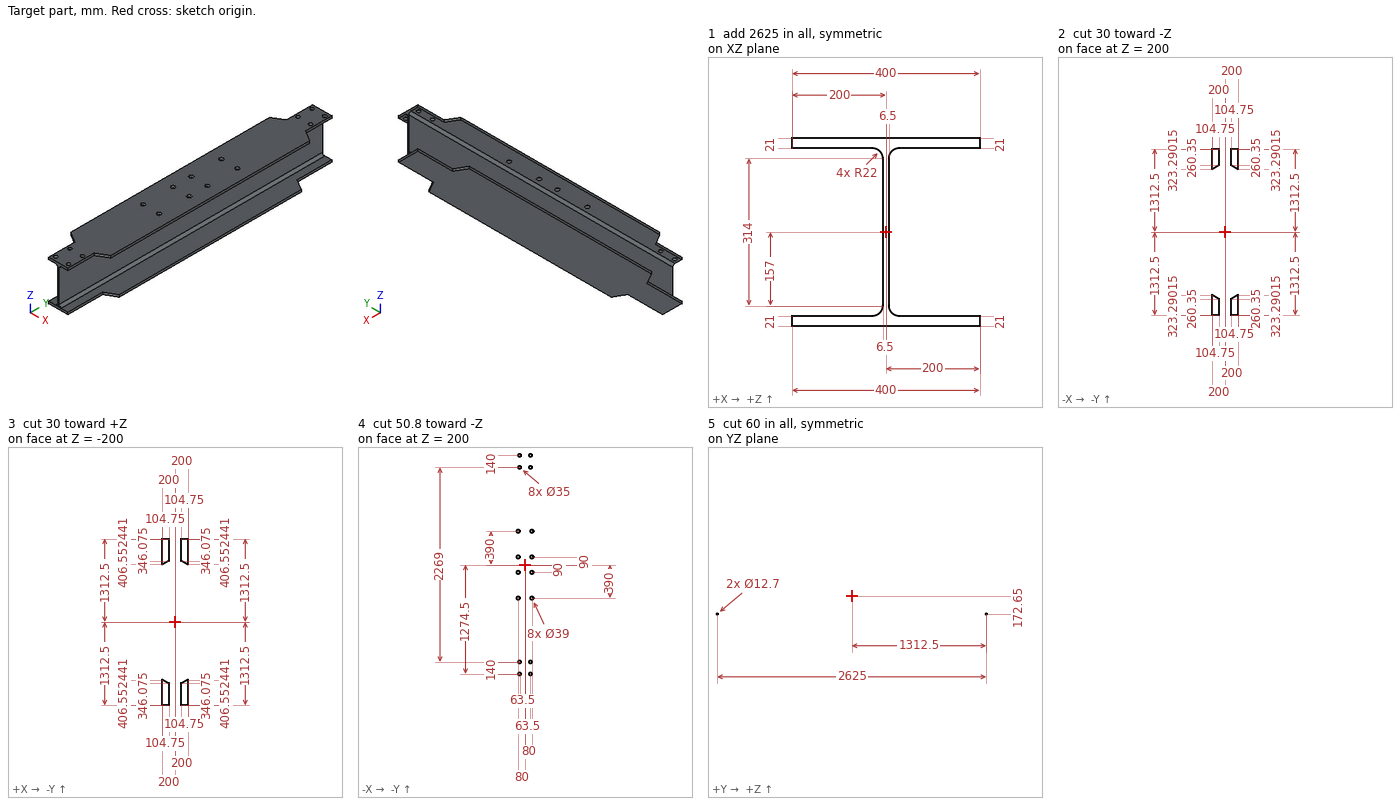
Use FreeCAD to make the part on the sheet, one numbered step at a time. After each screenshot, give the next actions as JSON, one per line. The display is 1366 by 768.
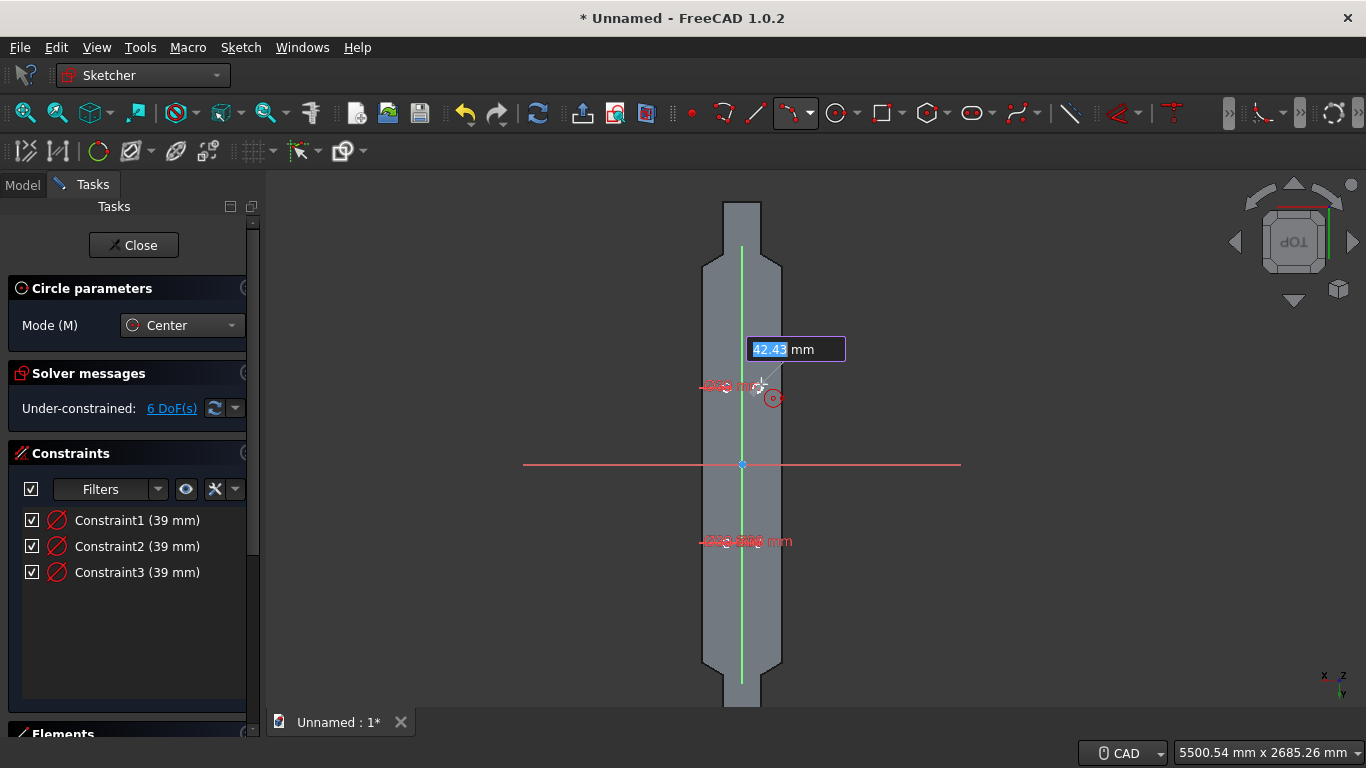
{"action": "type", "text": "39"}
{"action": "key", "text": "Return"}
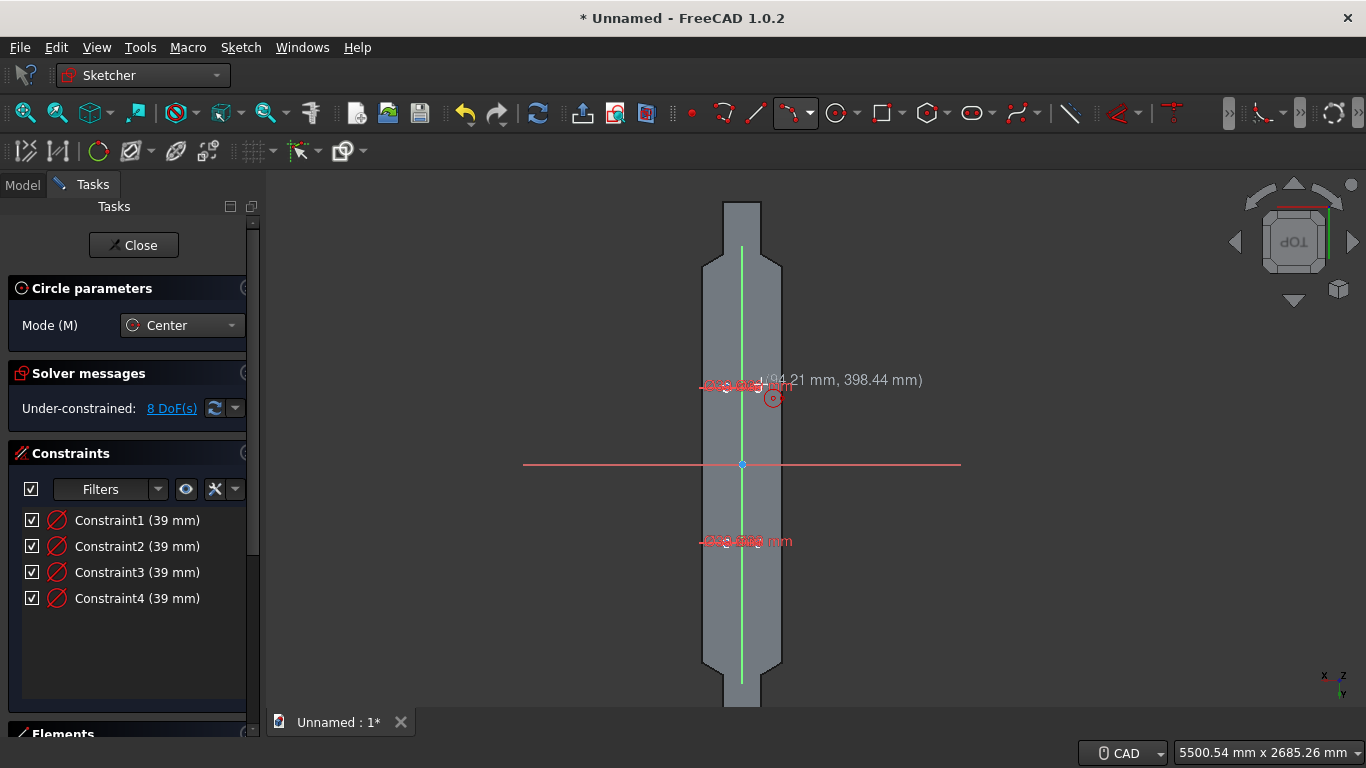
{"action": "scroll", "coordinate": [758, 385], "scroll_direction": "down", "scroll_amount": 2}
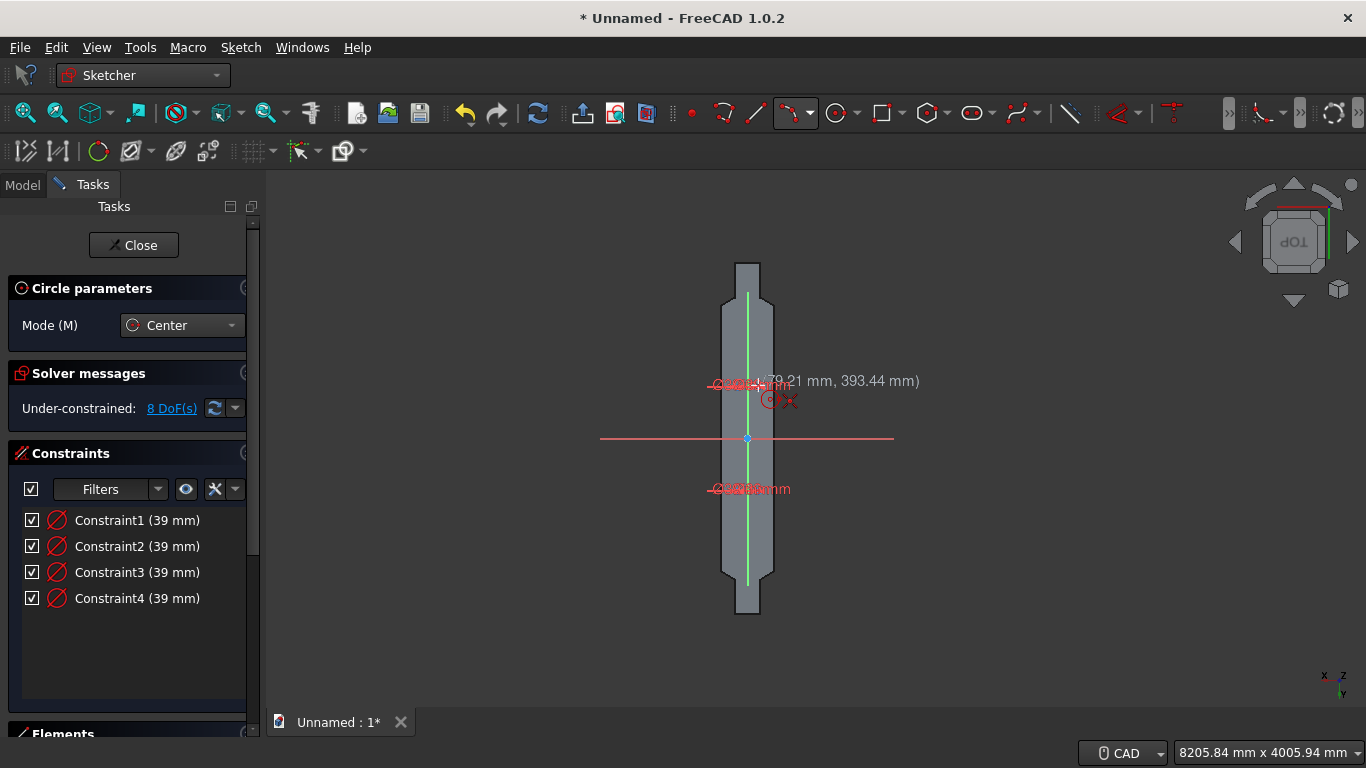
{"action": "scroll", "coordinate": [739, 609], "scroll_direction": "up", "scroll_amount": 12}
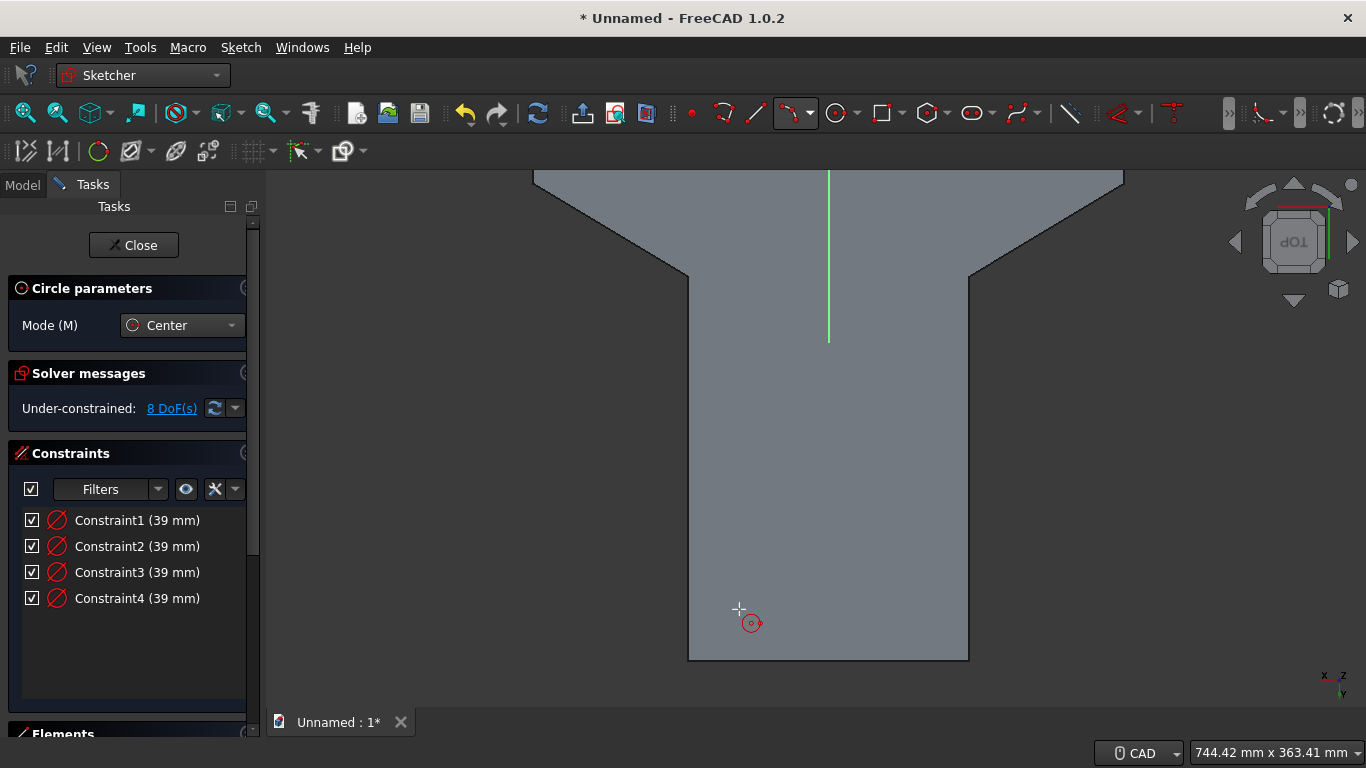
{"action": "scroll", "coordinate": [739, 610], "scroll_direction": "down", "scroll_amount": 12}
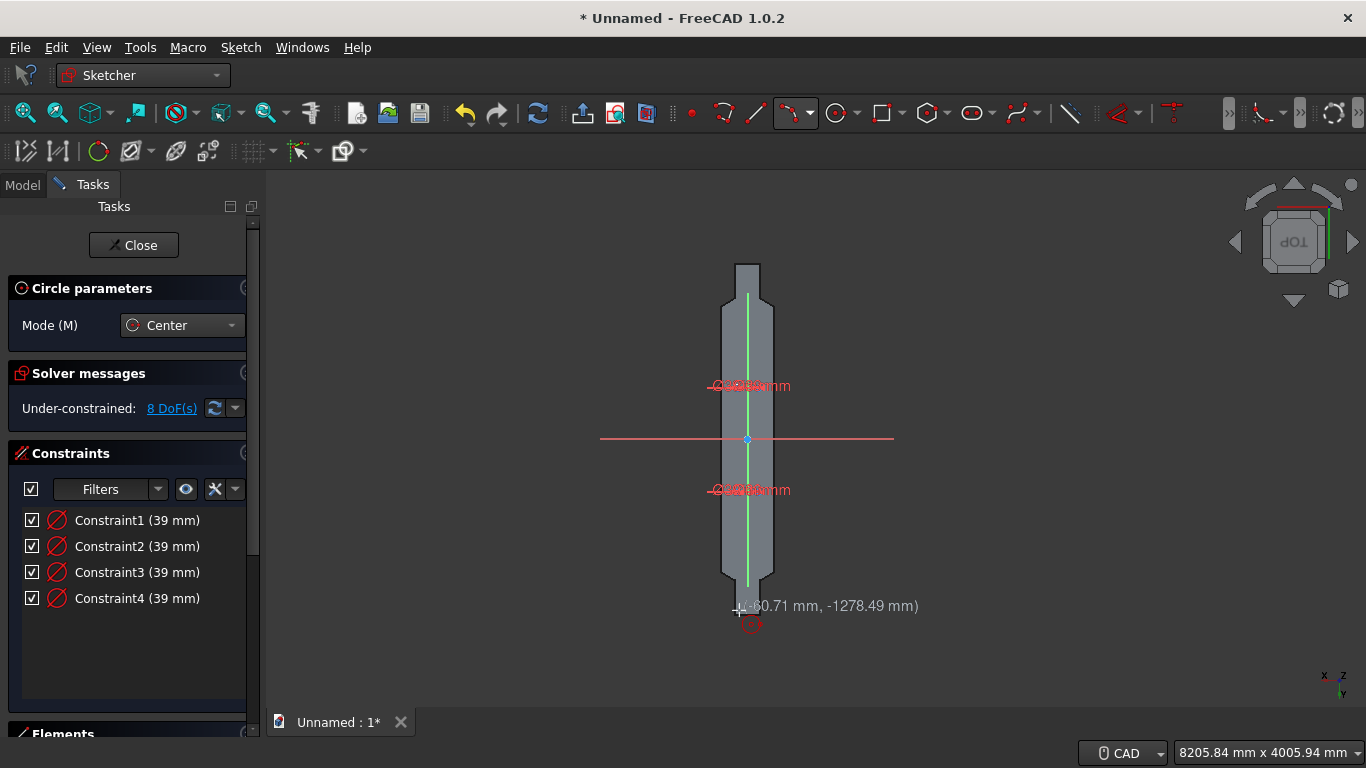
{"action": "scroll", "coordinate": [739, 610], "scroll_direction": "up", "scroll_amount": 4}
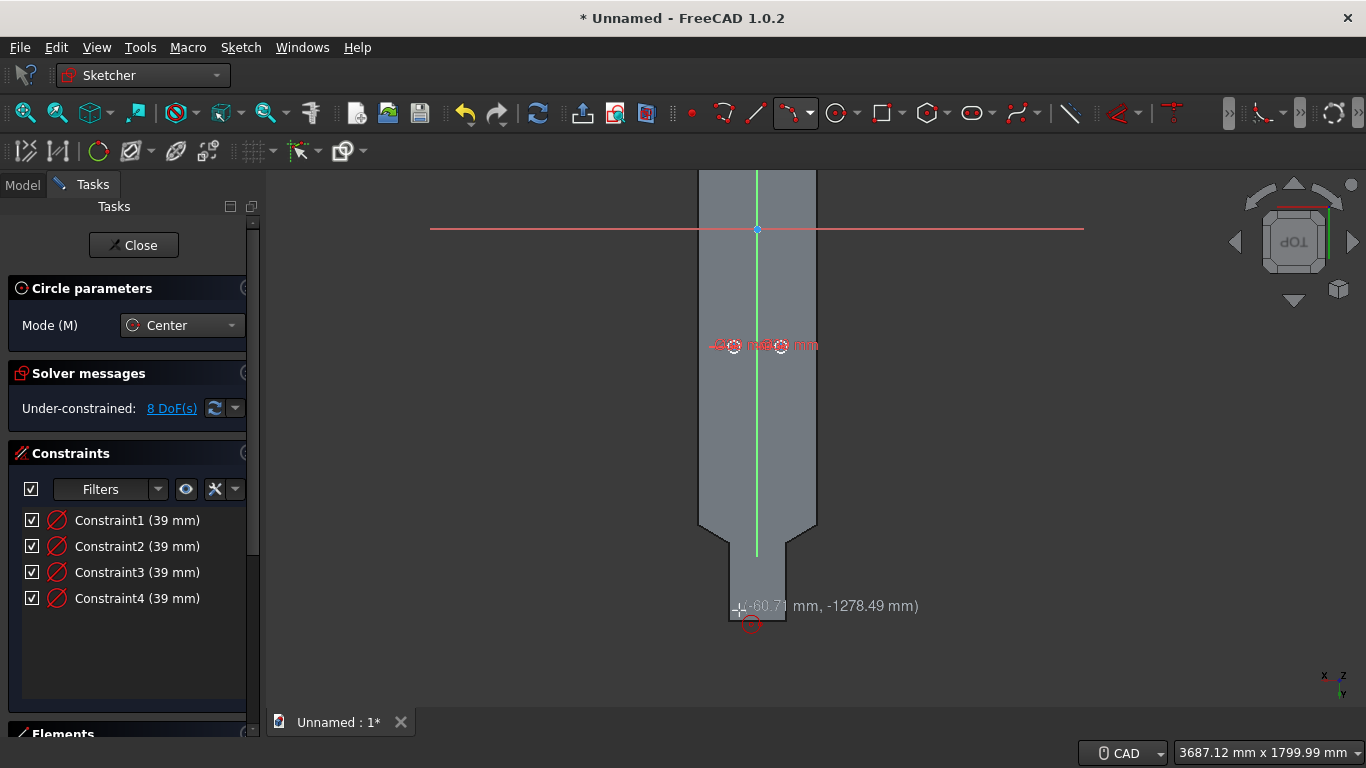
{"action": "left_click", "coordinate": [739, 610]}
{"action": "mouse_move", "coordinate": [742, 606]}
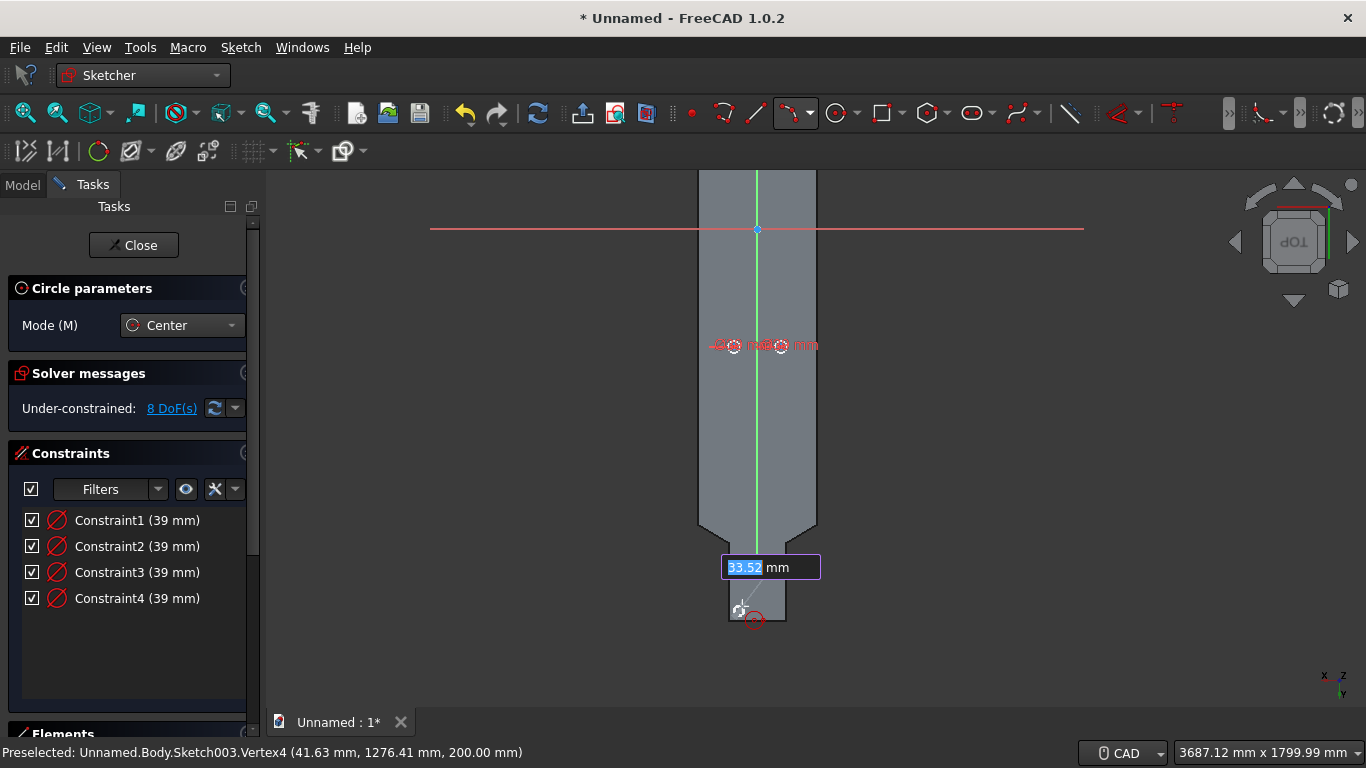
{"action": "type", "text": "35"}
{"action": "key", "text": "Return"}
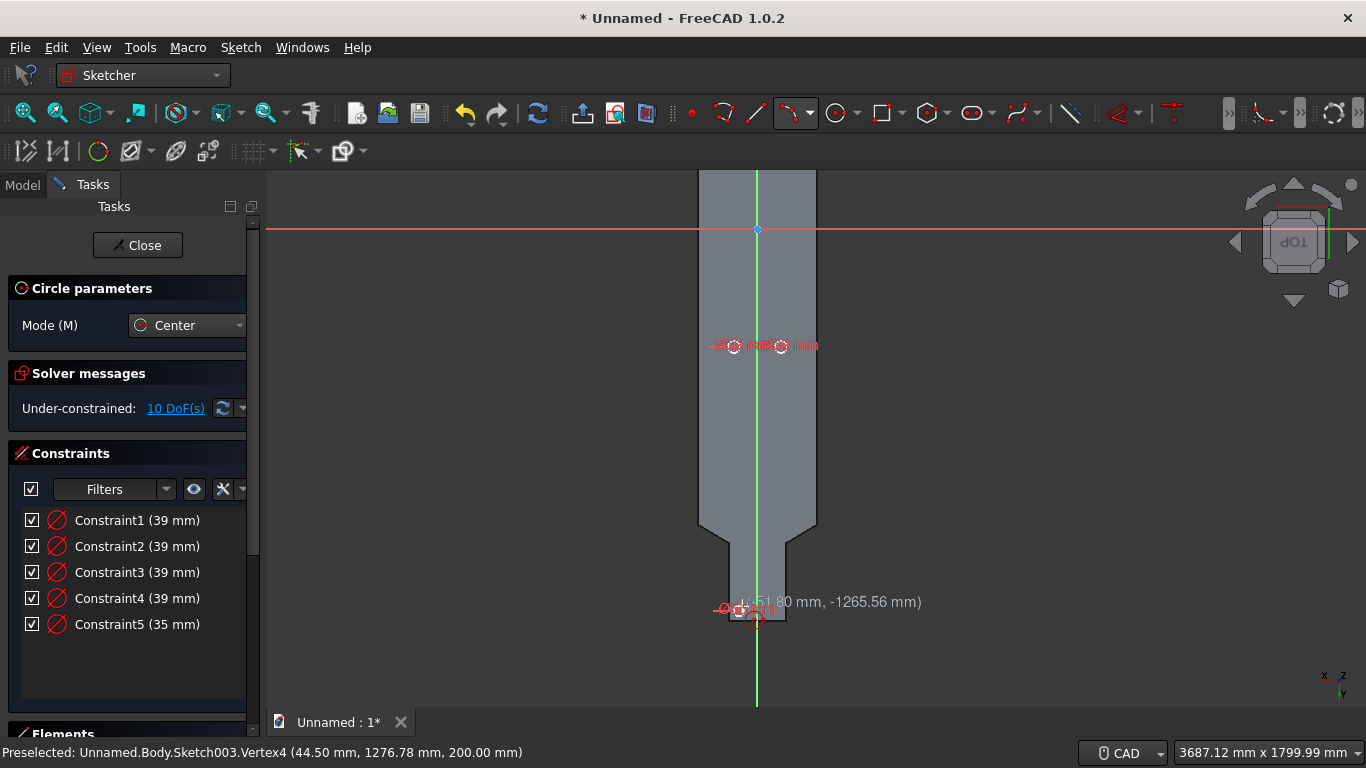
{"action": "scroll", "coordinate": [739, 568], "scroll_direction": "up", "scroll_amount": 8}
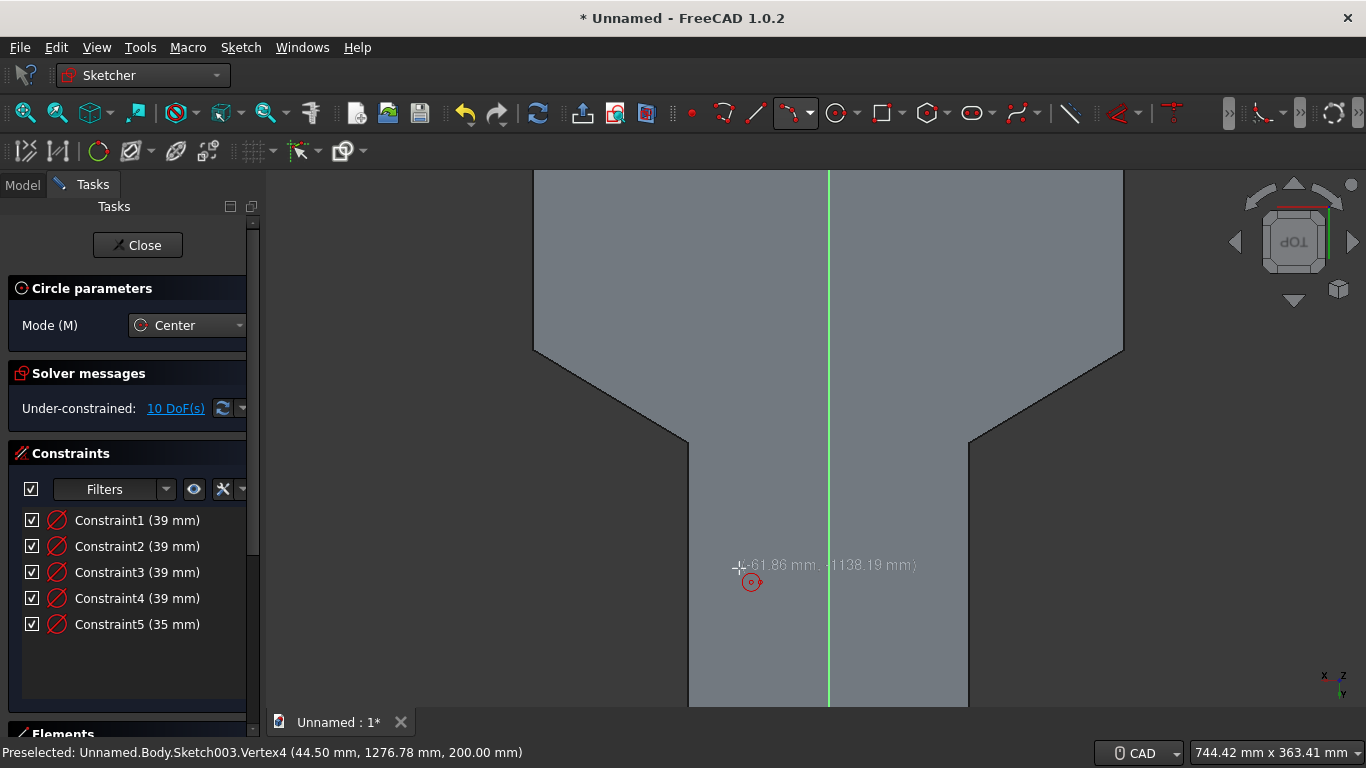
{"action": "scroll", "coordinate": [739, 593], "scroll_direction": "down", "scroll_amount": 12}